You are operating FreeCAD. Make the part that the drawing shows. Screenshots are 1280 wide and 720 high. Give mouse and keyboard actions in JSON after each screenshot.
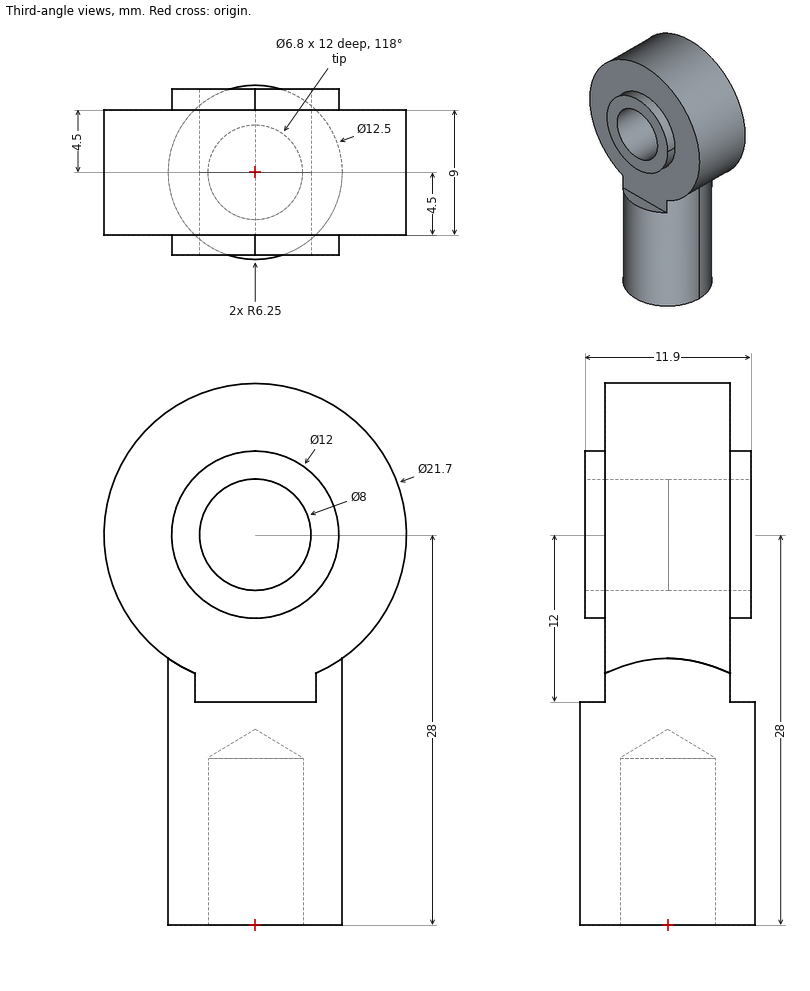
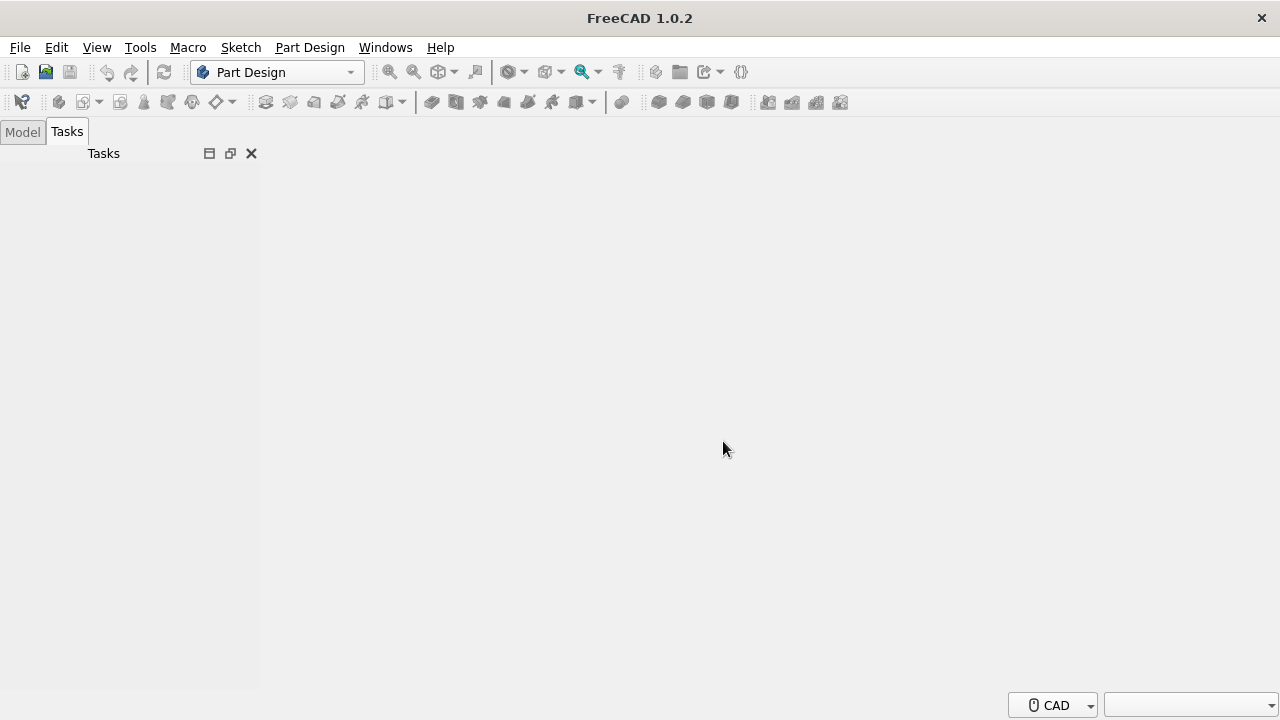
{"action": "key", "text": "ctrl+n"}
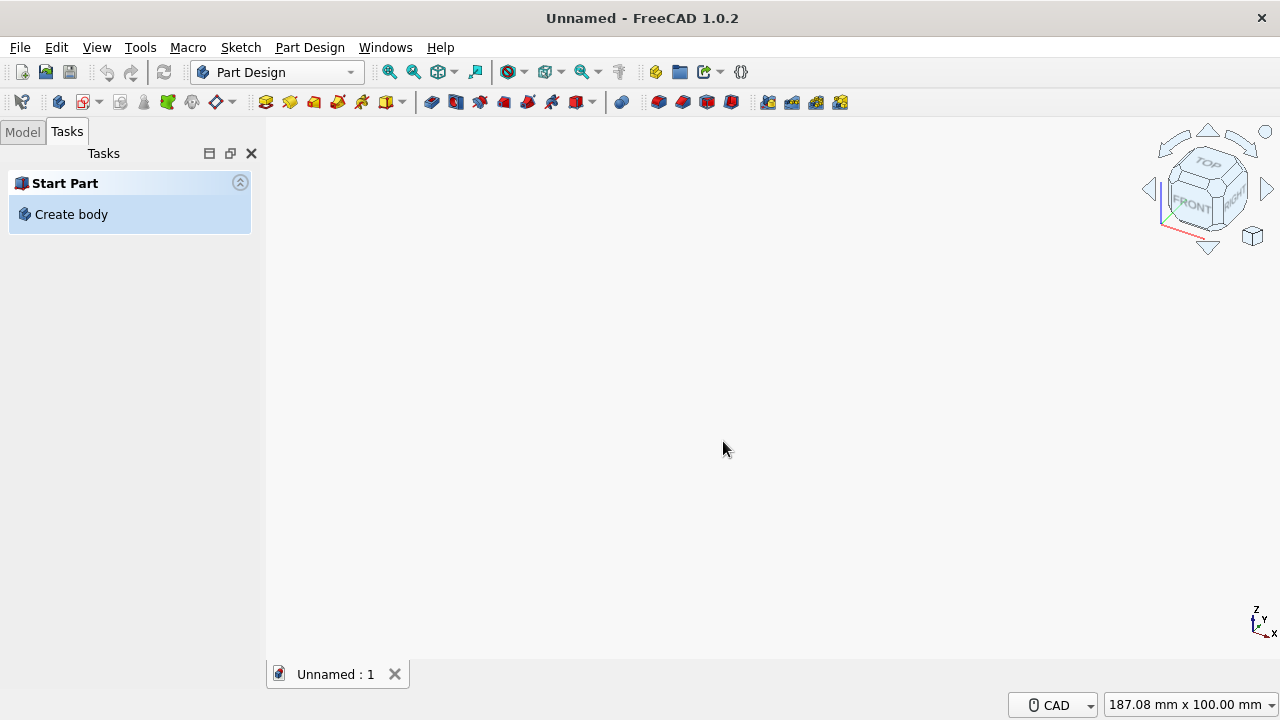
{"action": "left_click", "coordinate": [84, 102]}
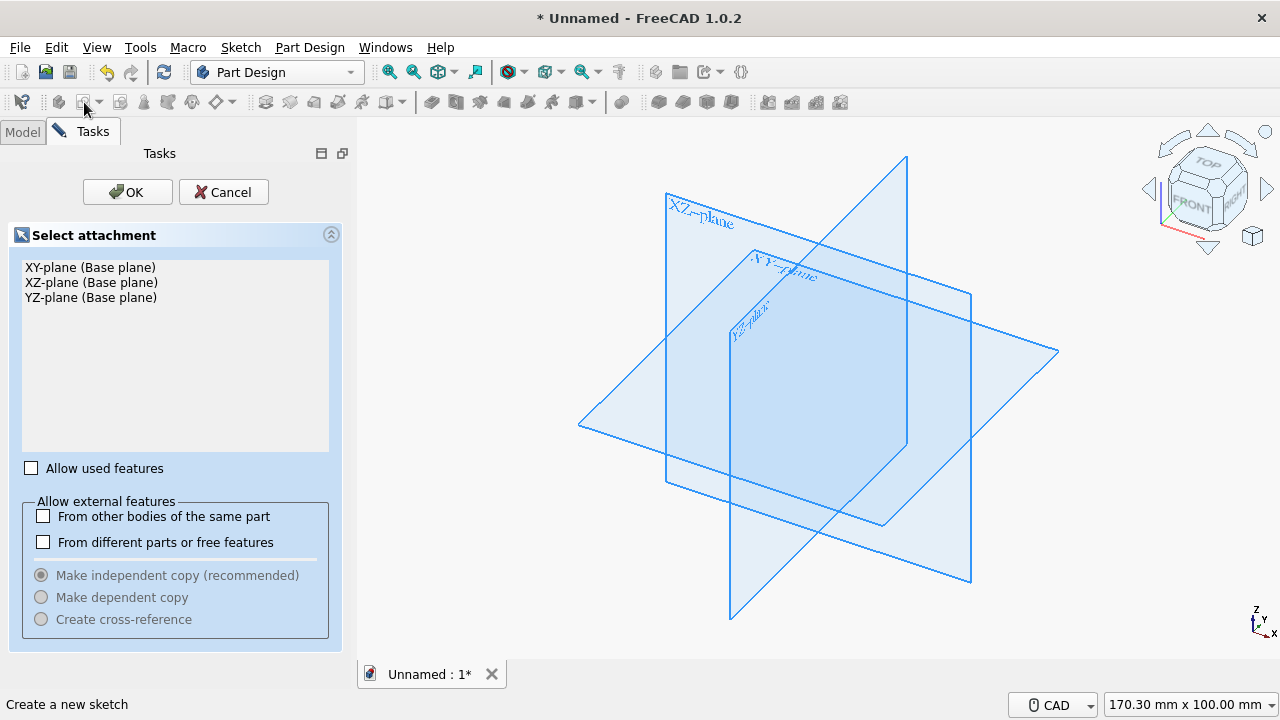
{"action": "left_click", "coordinate": [82, 268]}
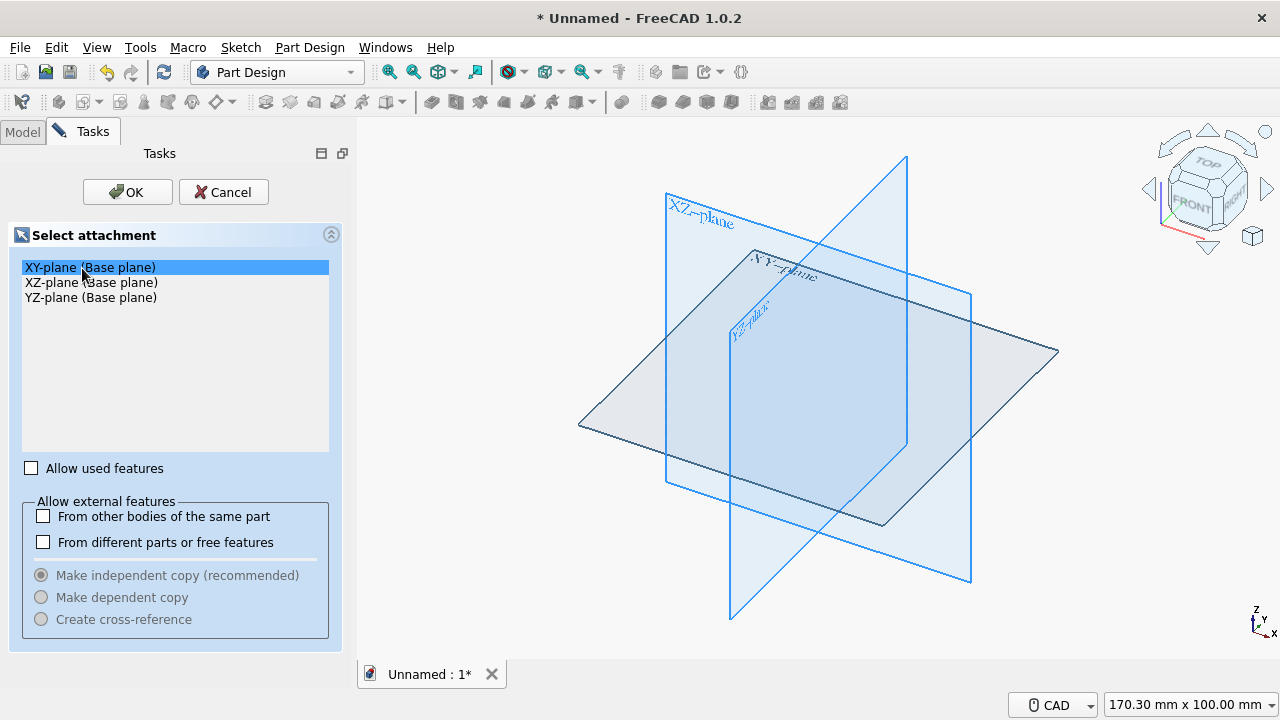
{"action": "left_click", "coordinate": [128, 192]}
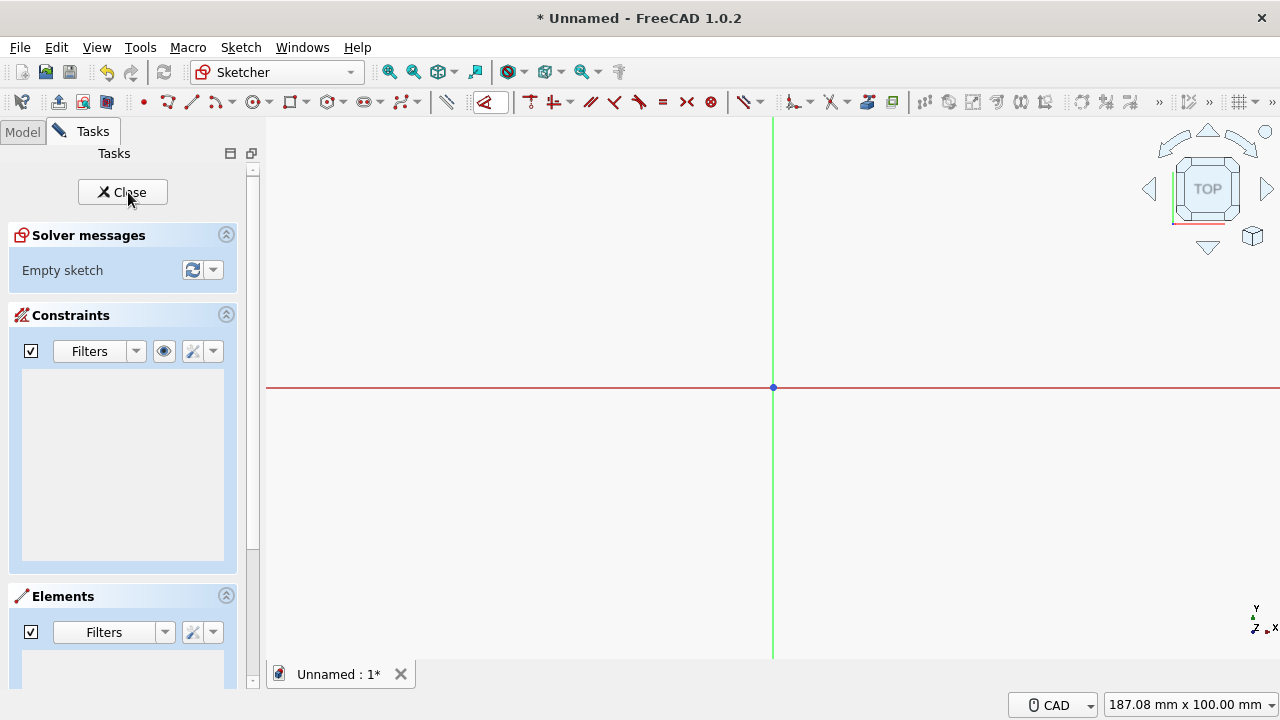
{"action": "scroll", "coordinate": [790, 388], "scroll_direction": "up", "scroll_amount": 8}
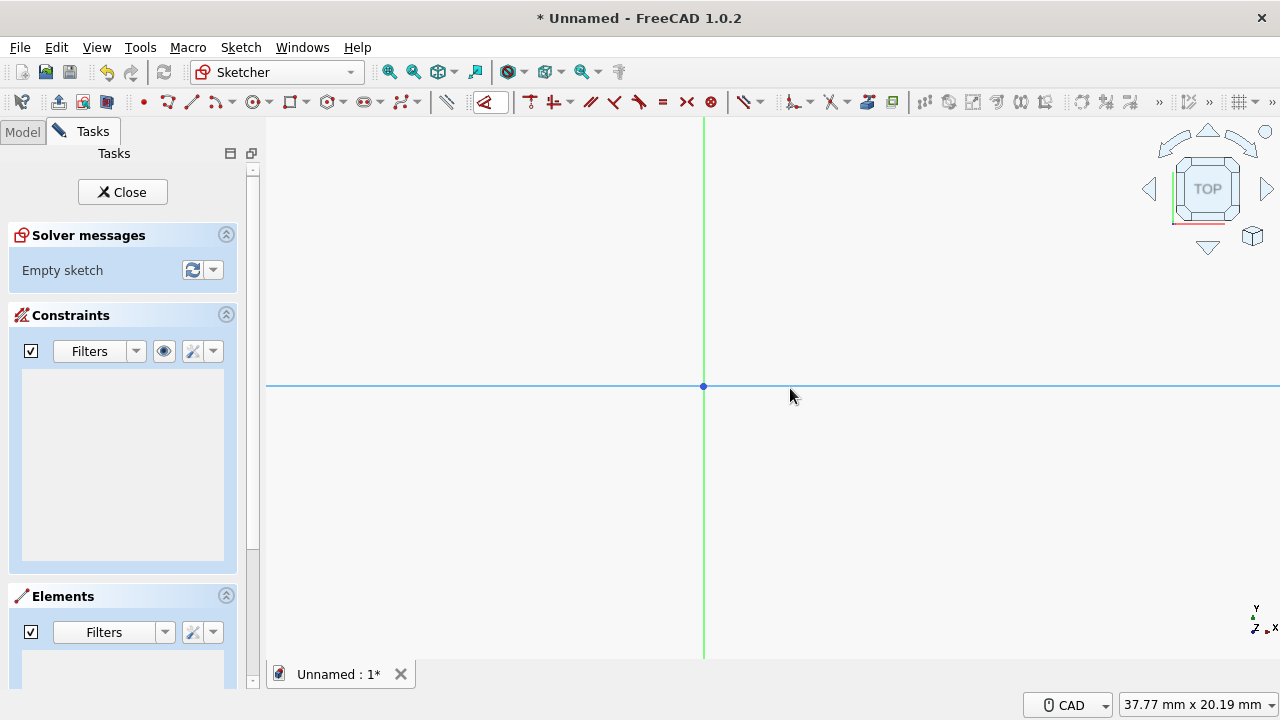
{"action": "left_click", "coordinate": [254, 102]}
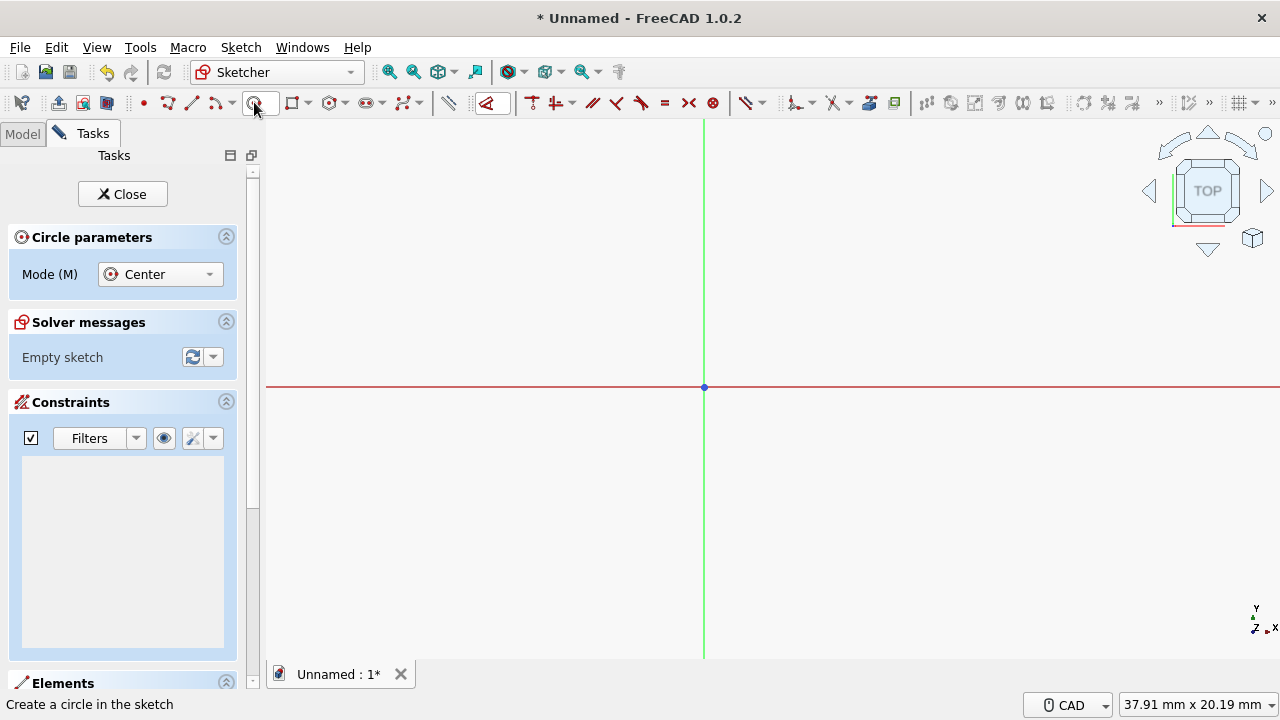
{"action": "left_click", "coordinate": [704, 387]}
{"action": "left_click", "coordinate": [822, 269]}
{"action": "key", "text": "Escape"}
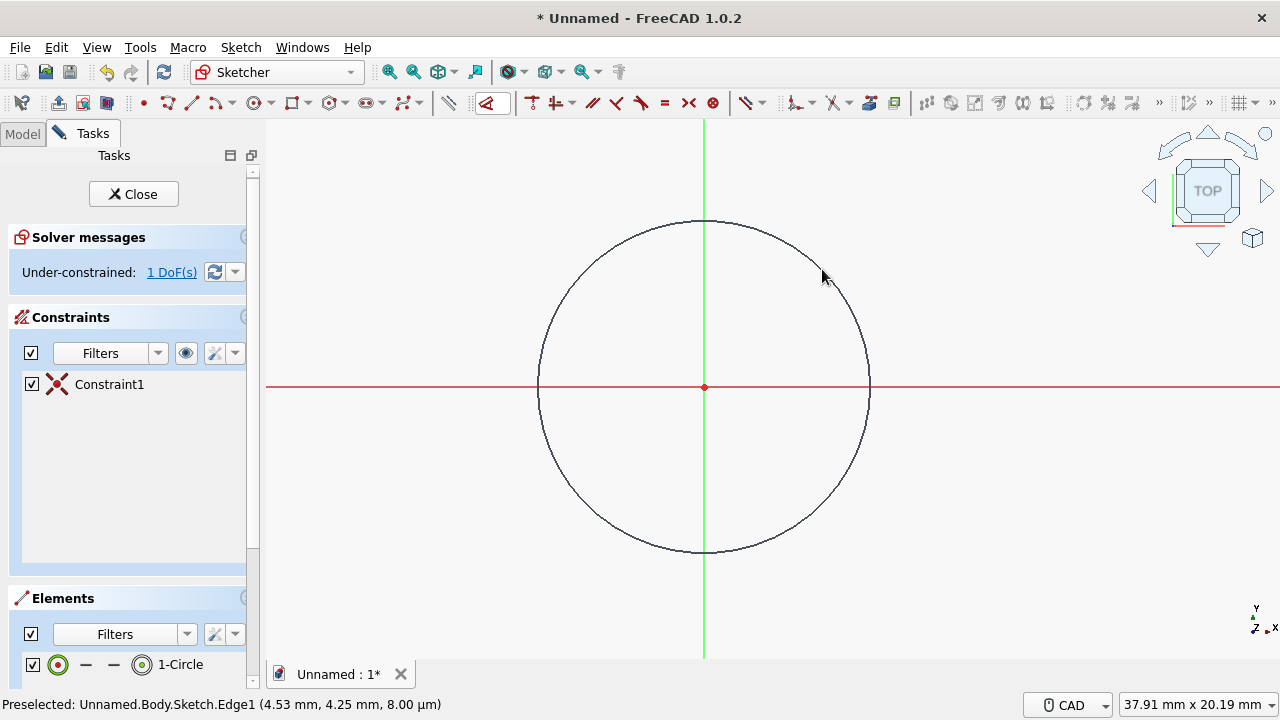
{"action": "left_click", "coordinate": [821, 269]}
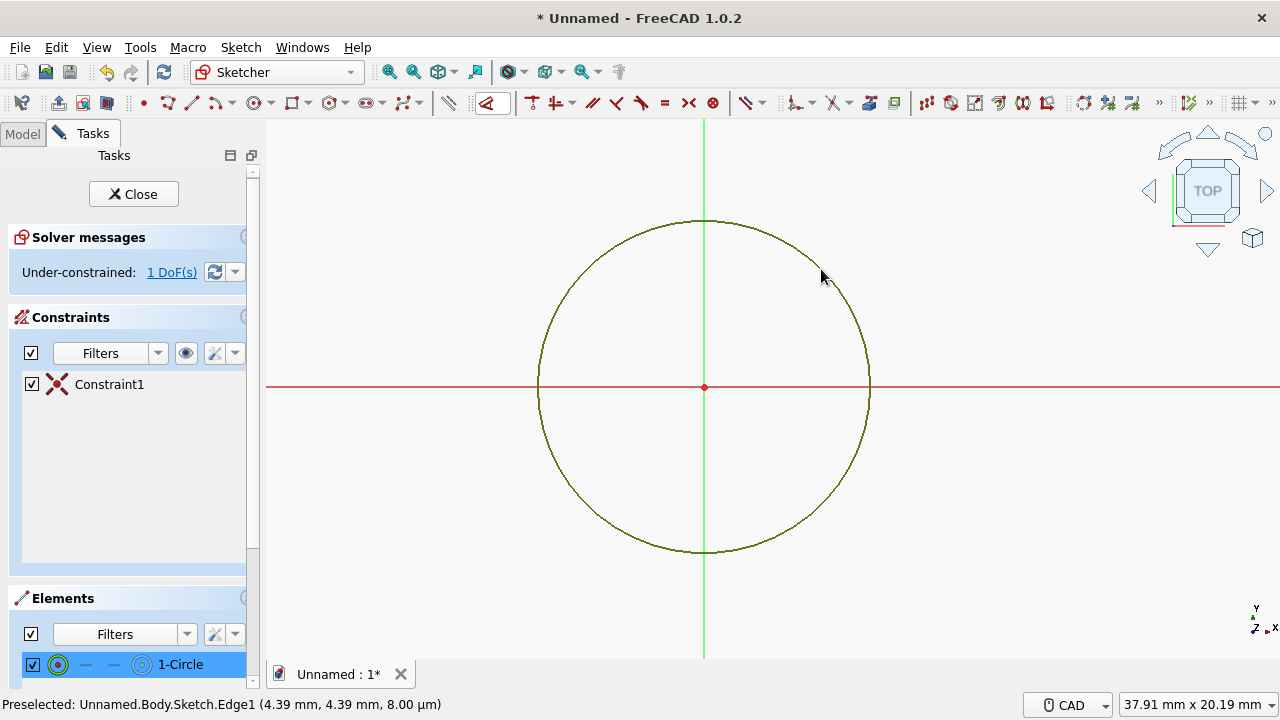
{"action": "key", "text": "k o"}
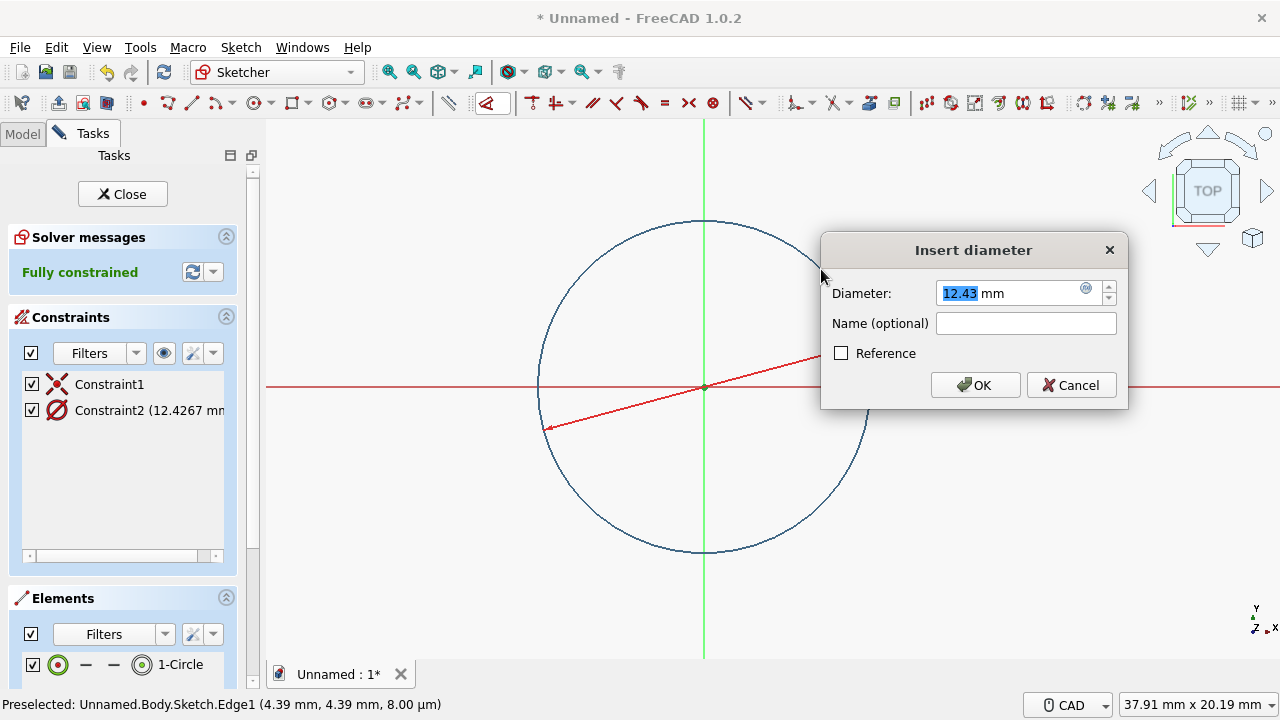
{"action": "type", "text": "12.5"}
{"action": "key", "text": "Return"}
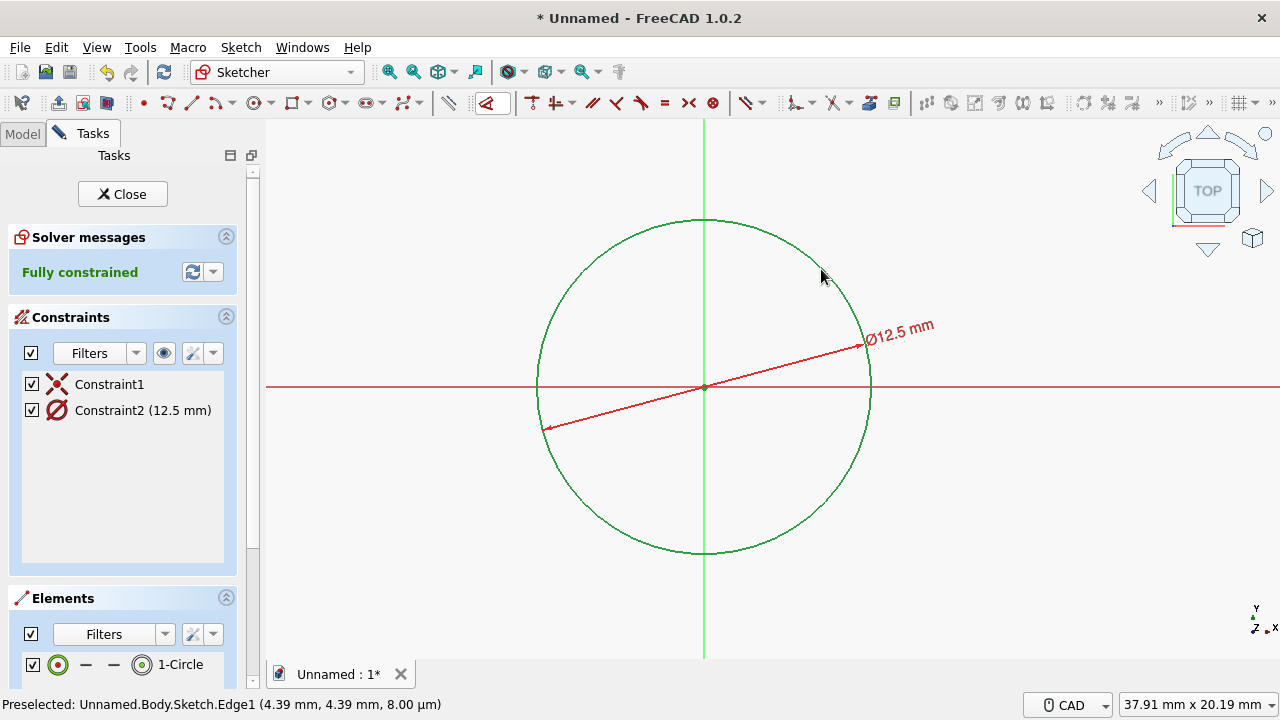
{"action": "left_click", "coordinate": [123, 194]}